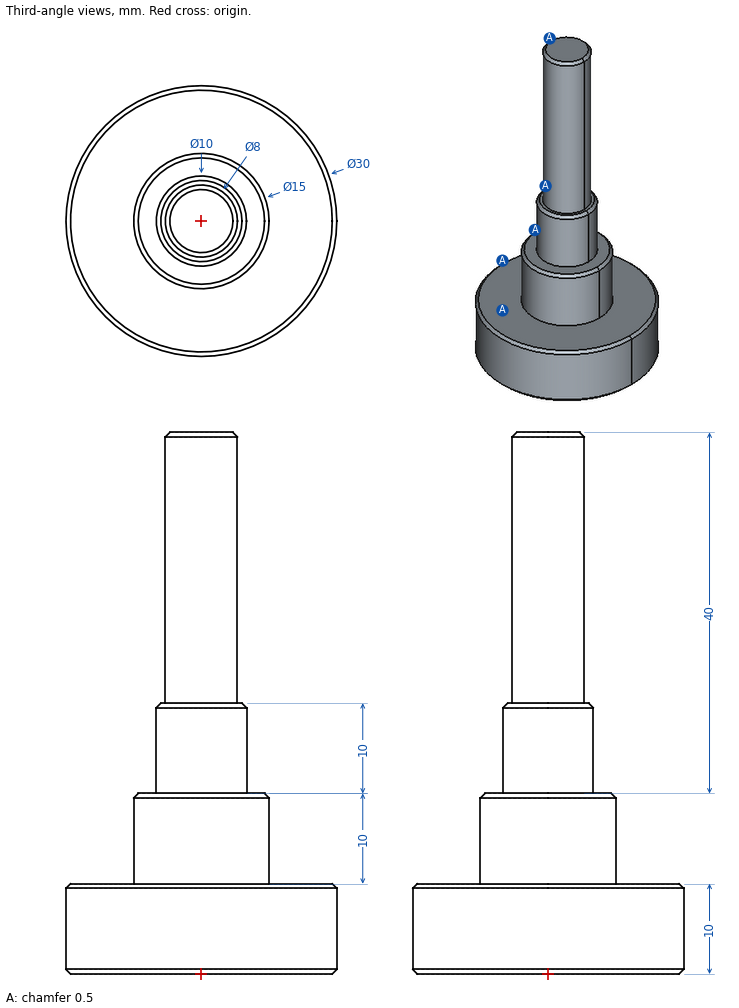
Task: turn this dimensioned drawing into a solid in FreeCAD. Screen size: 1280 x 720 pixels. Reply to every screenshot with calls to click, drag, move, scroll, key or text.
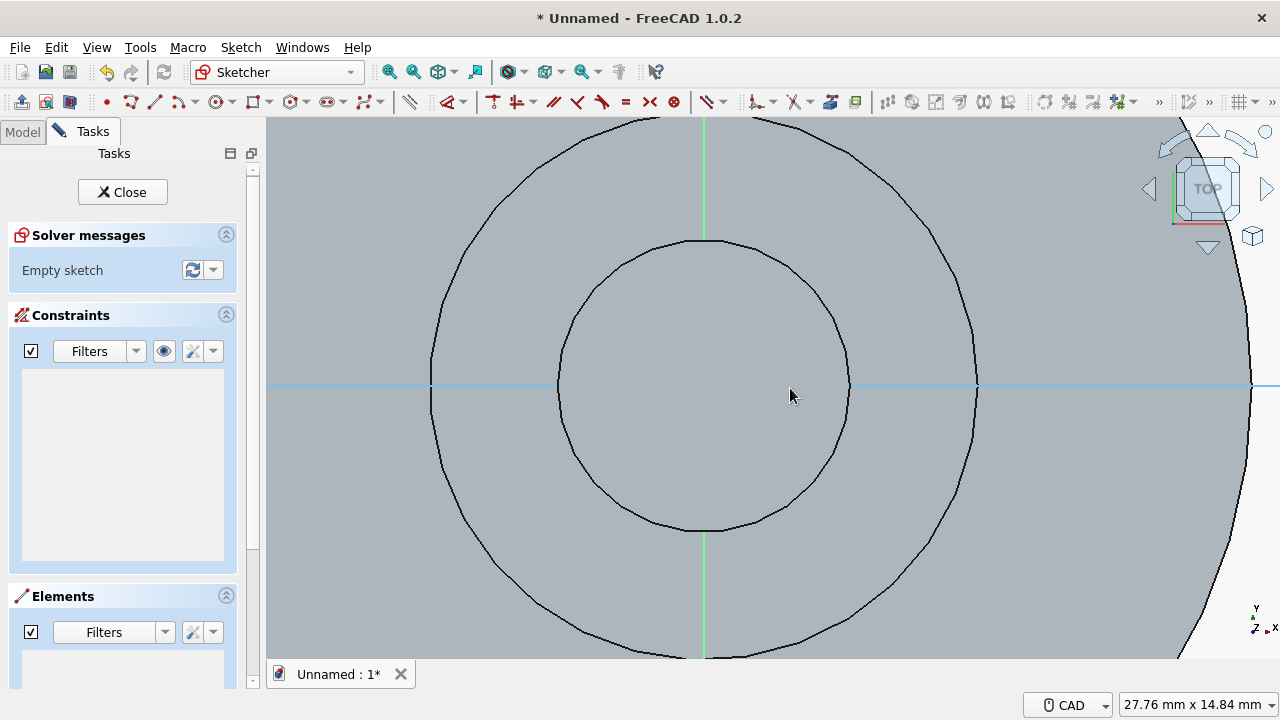
click(216, 102)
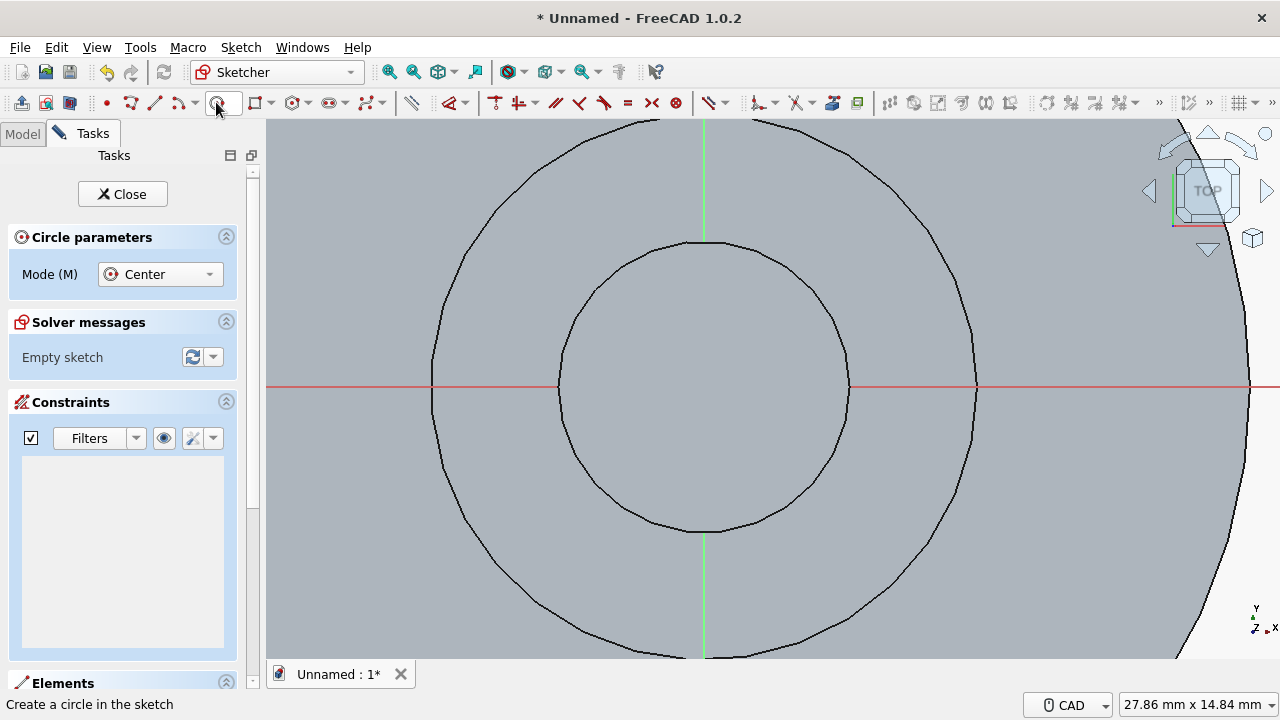
click(704, 387)
click(833, 258)
key(Escape)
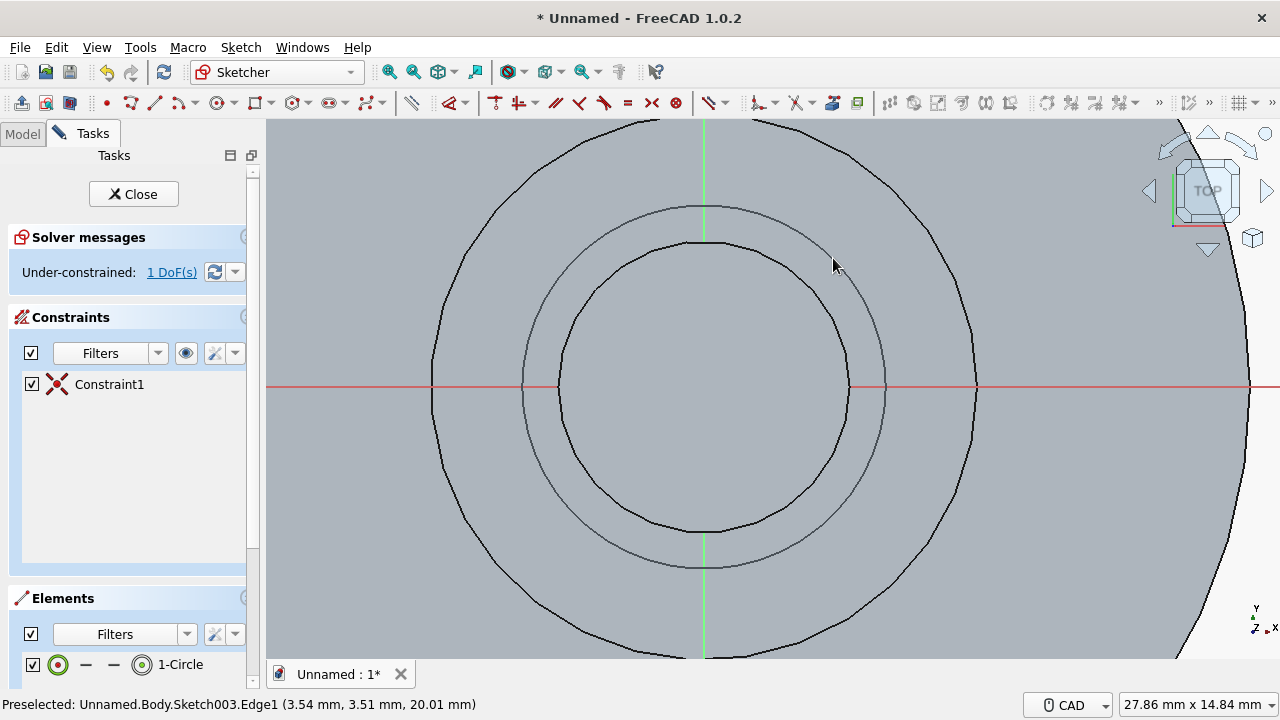
click(832, 258)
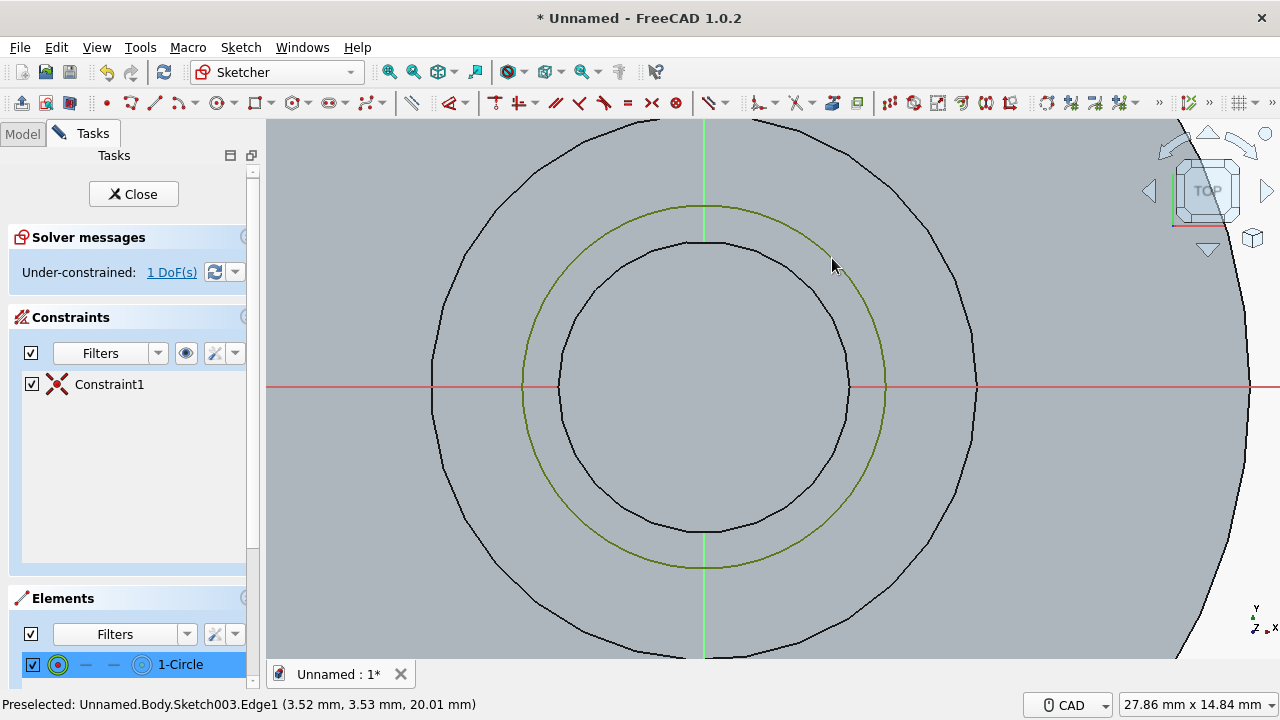
key(k)
key(o)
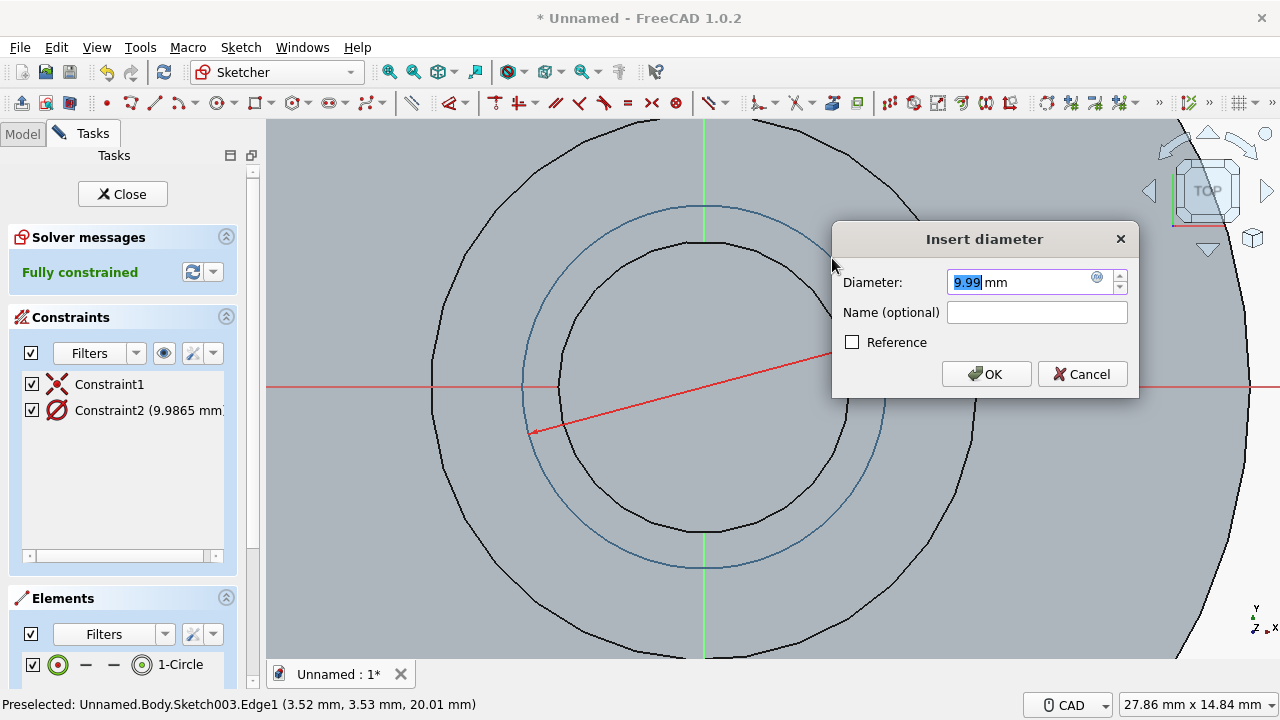
text(10)
key(Return)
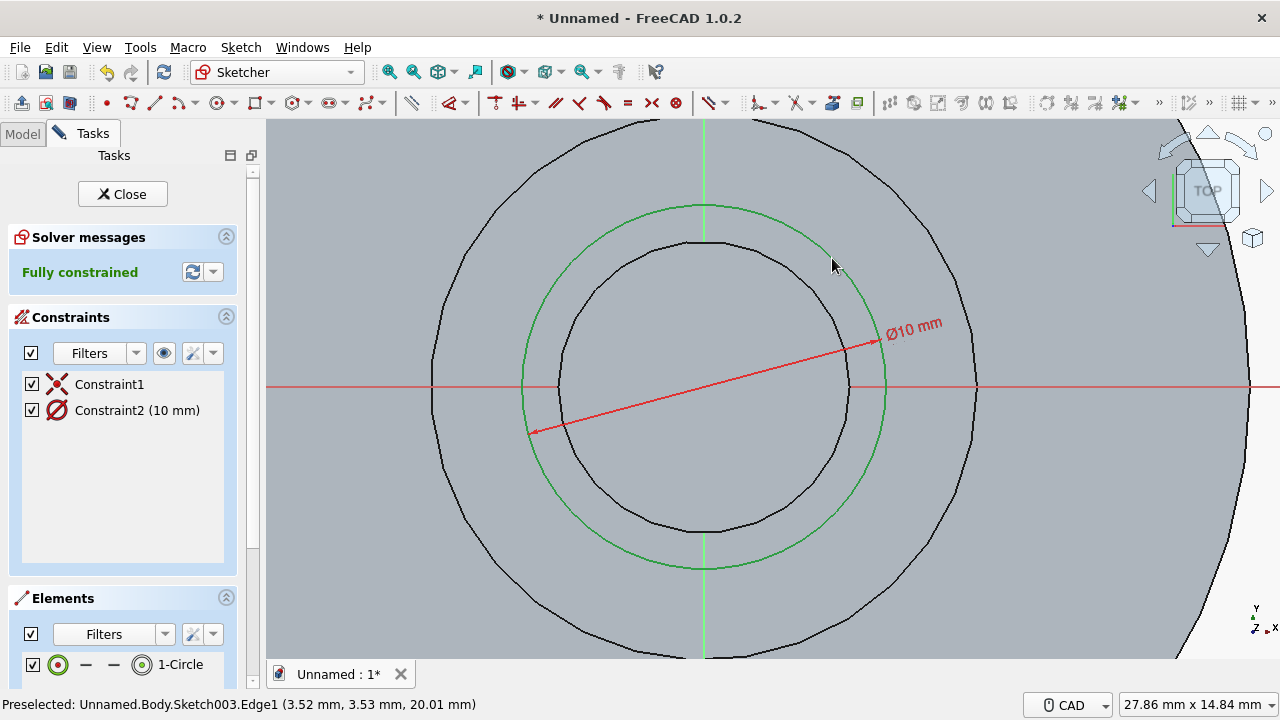
click(123, 194)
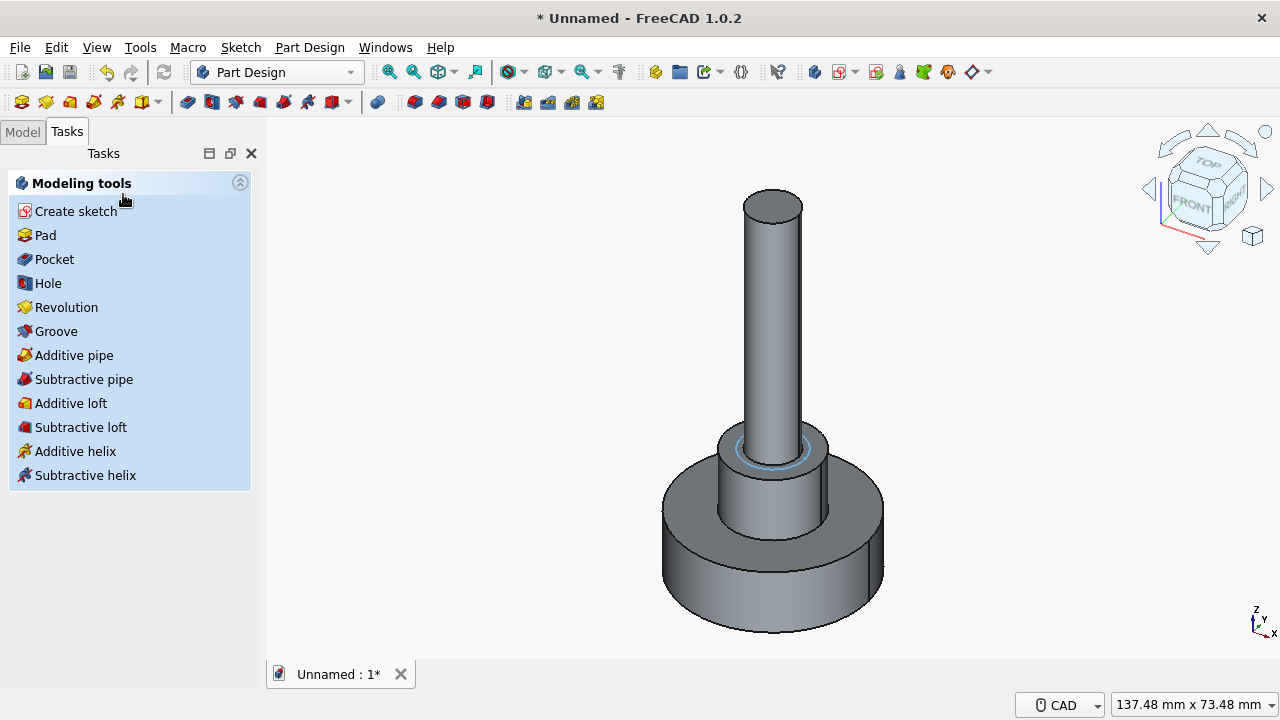
click(22, 102)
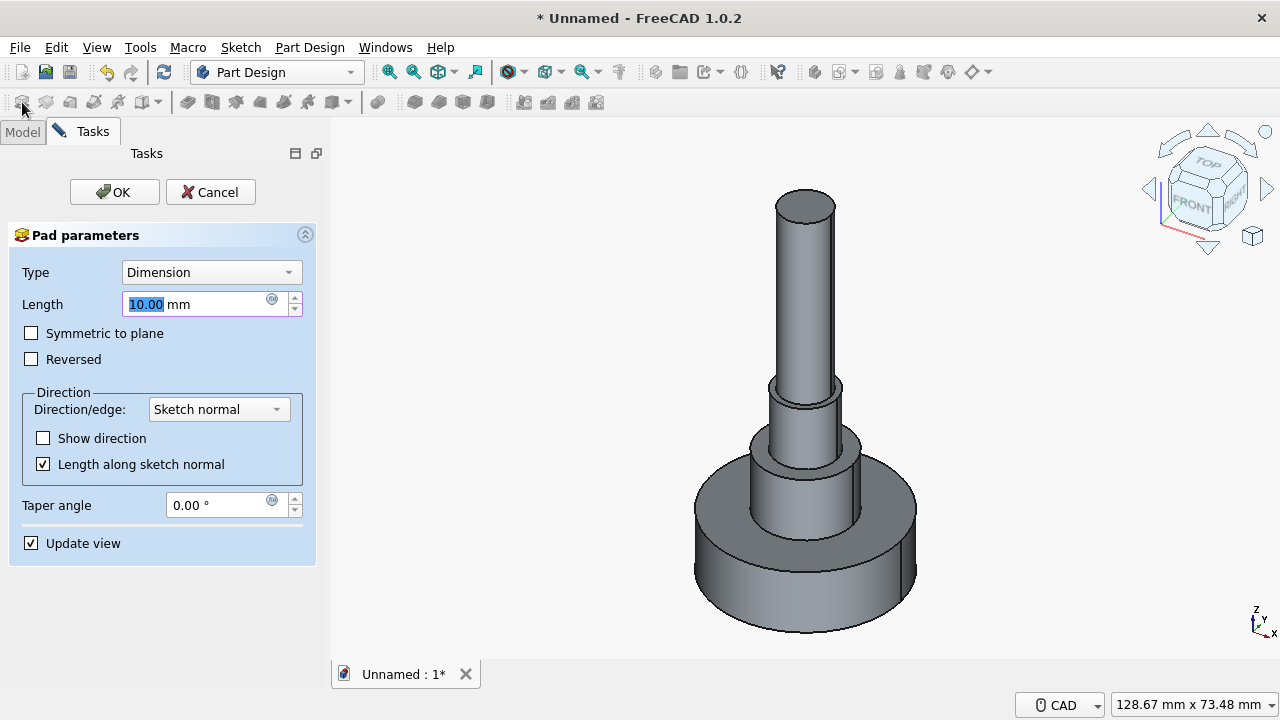
text(10)
key(Tab)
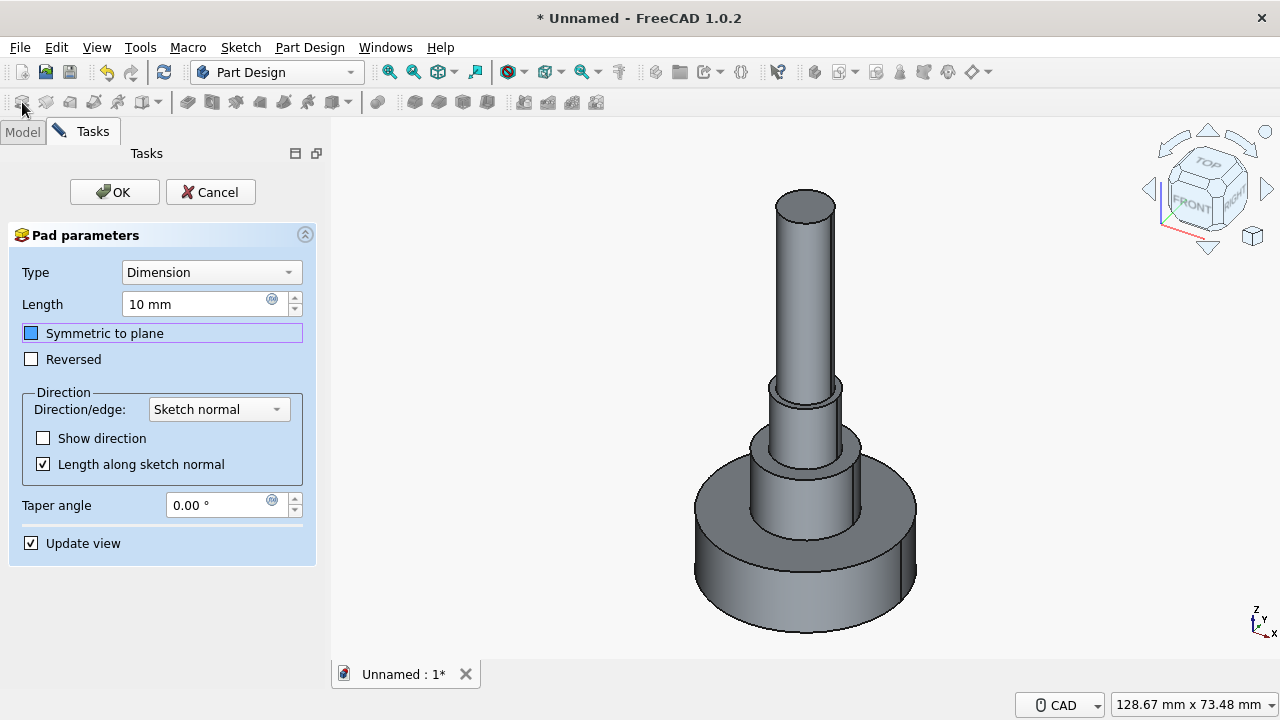
click(115, 192)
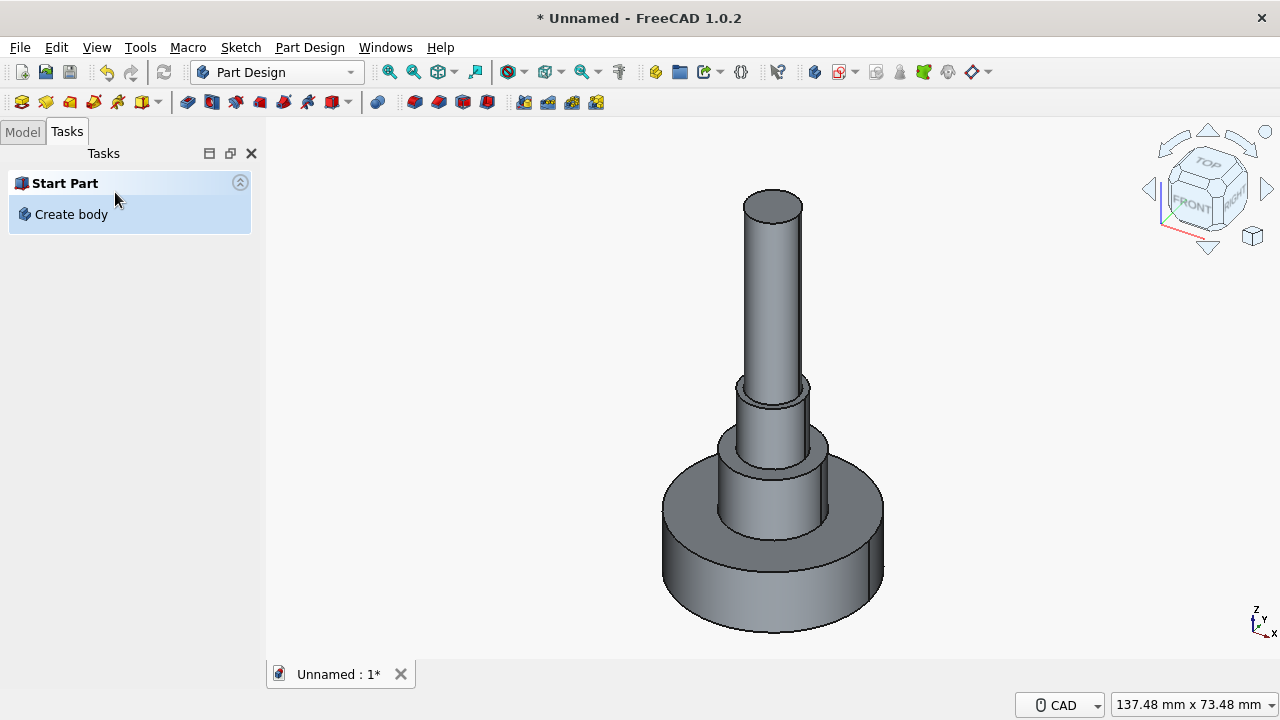
click(744, 208)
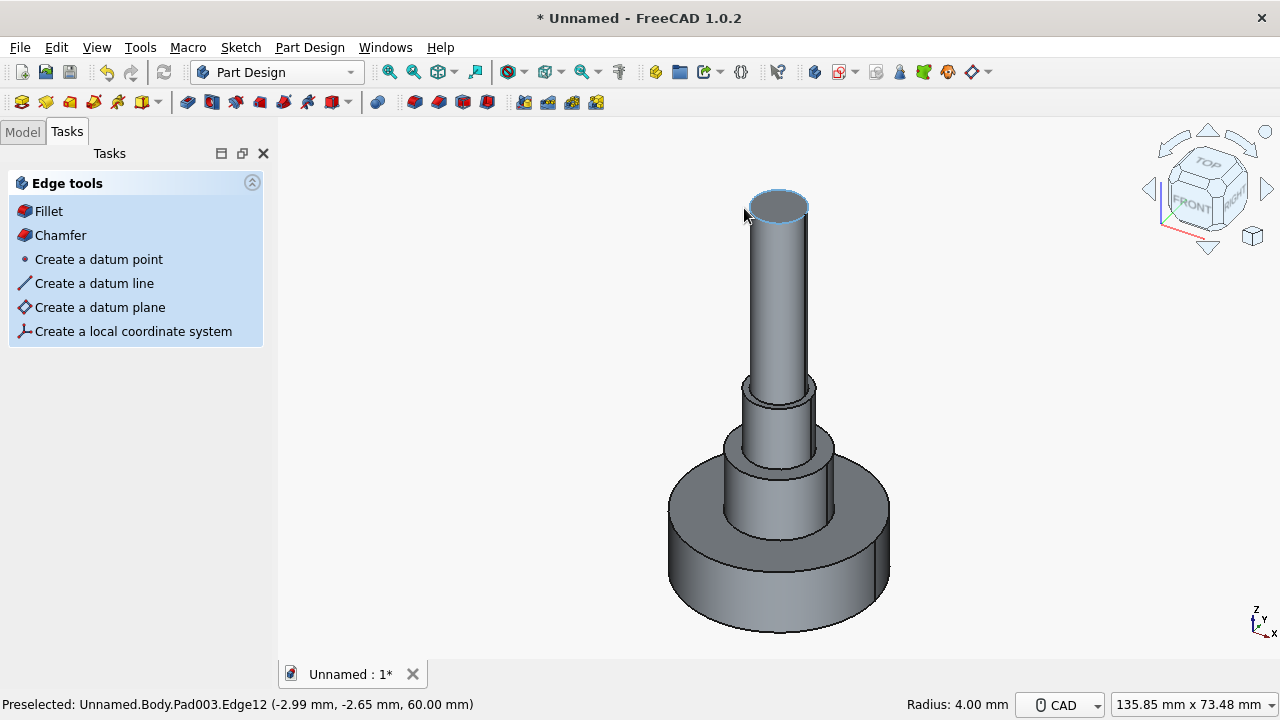
click(742, 389, ctrl)